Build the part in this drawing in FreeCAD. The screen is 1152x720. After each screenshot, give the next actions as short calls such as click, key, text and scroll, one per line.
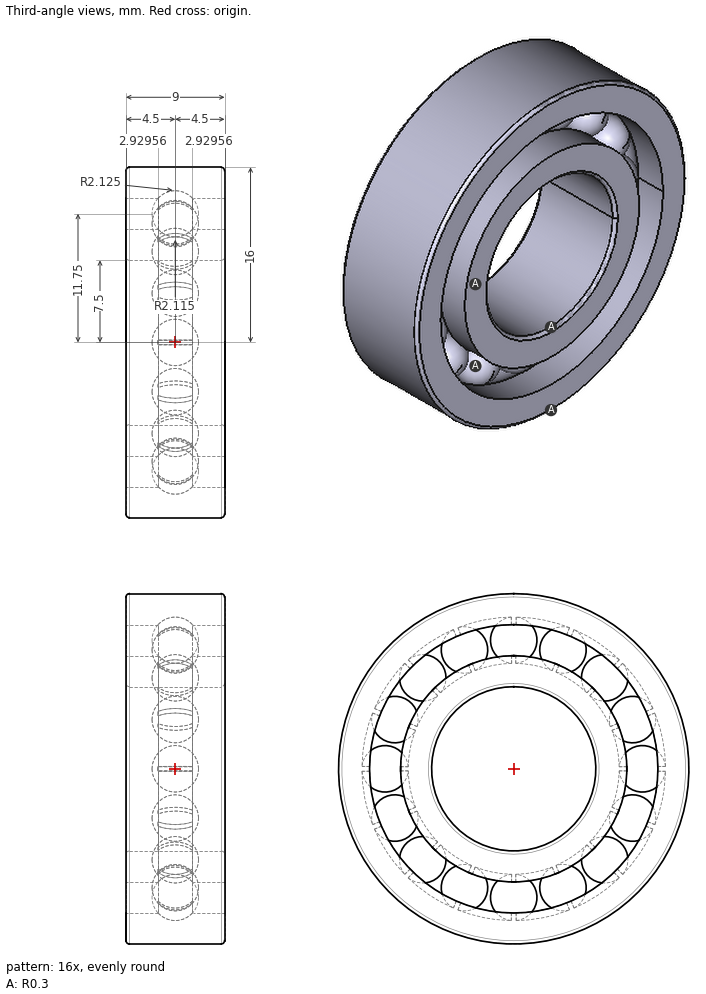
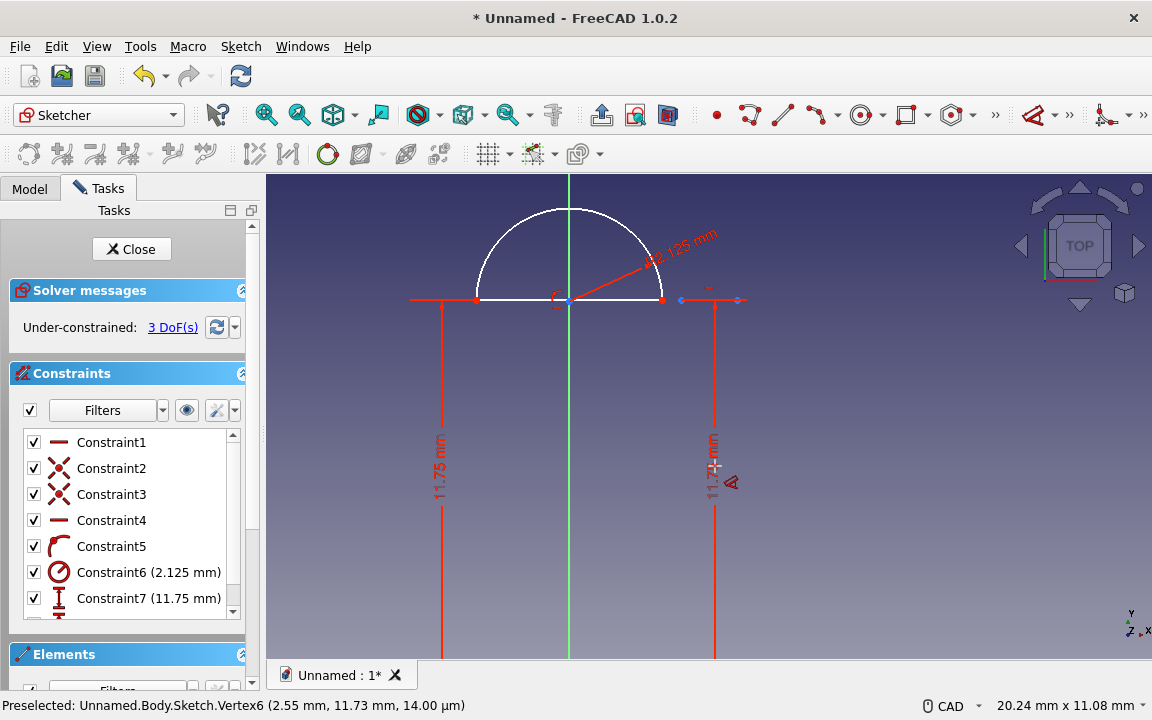
click(569, 302)
click(535, 466)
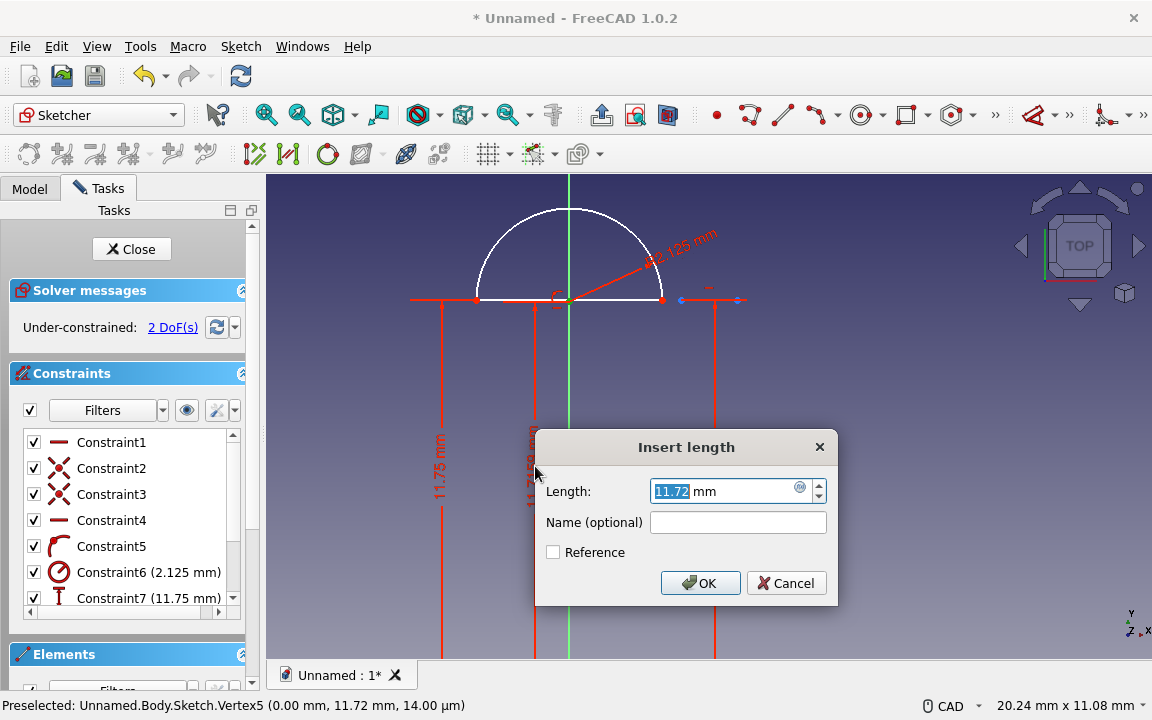
text(11.75)
key(Return)
key(Escape)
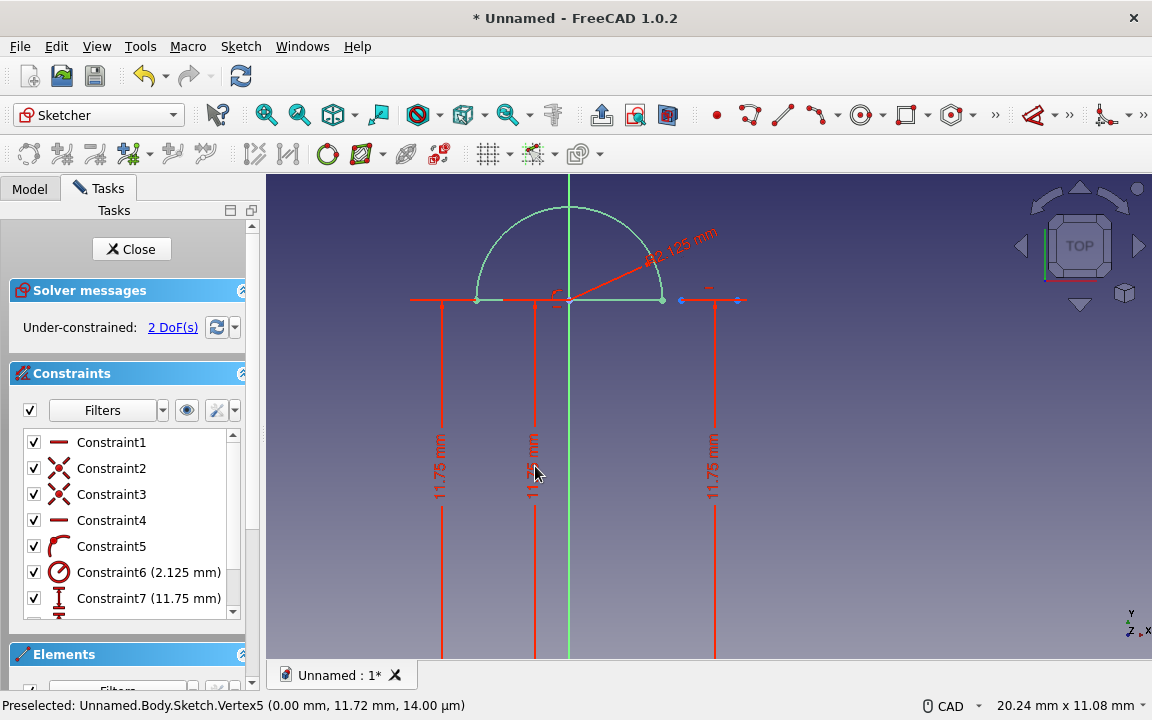
click(132, 249)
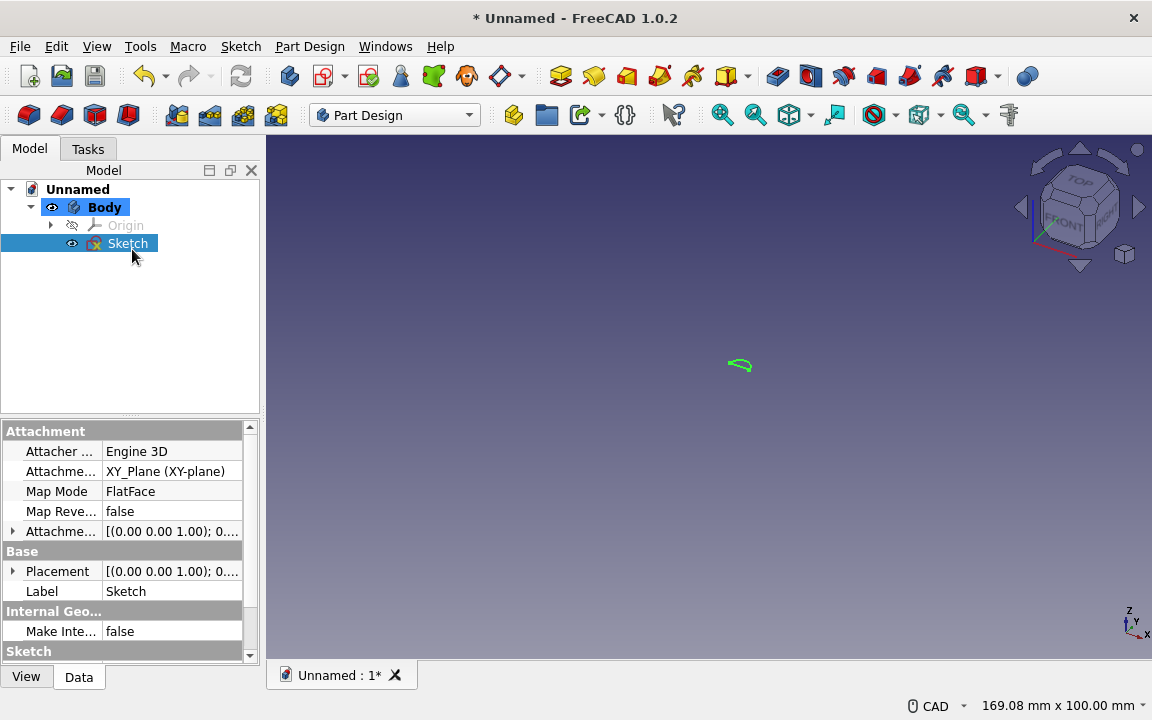
click(594, 76)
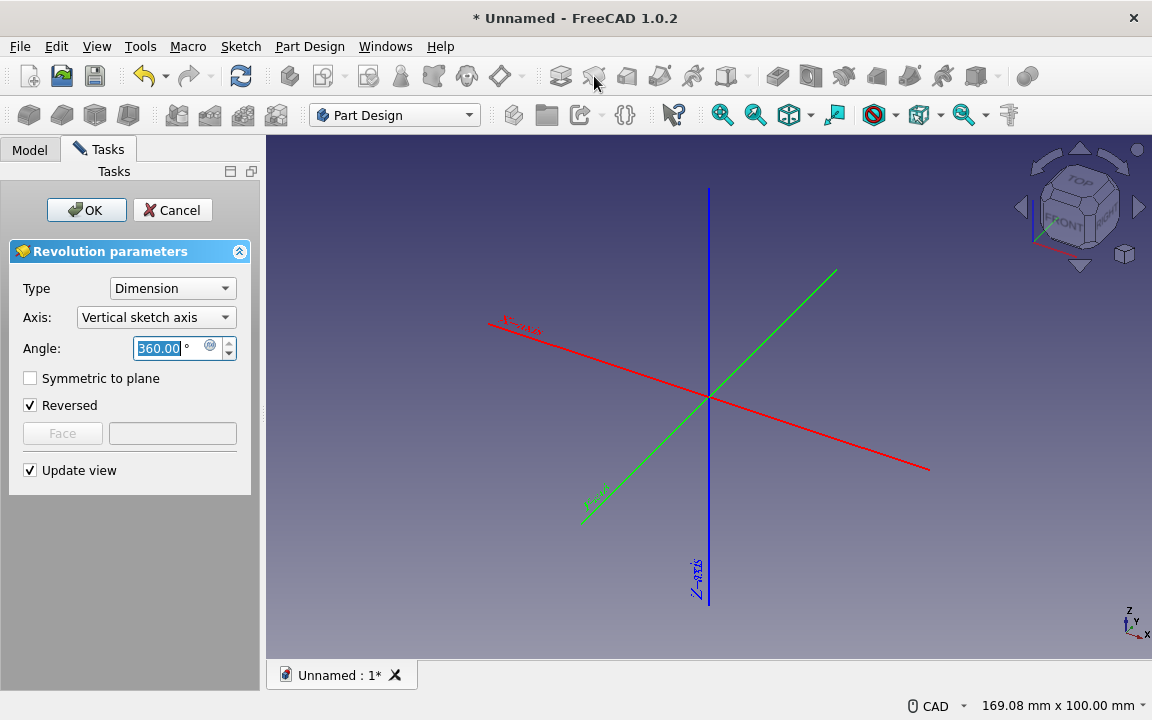
click(157, 318)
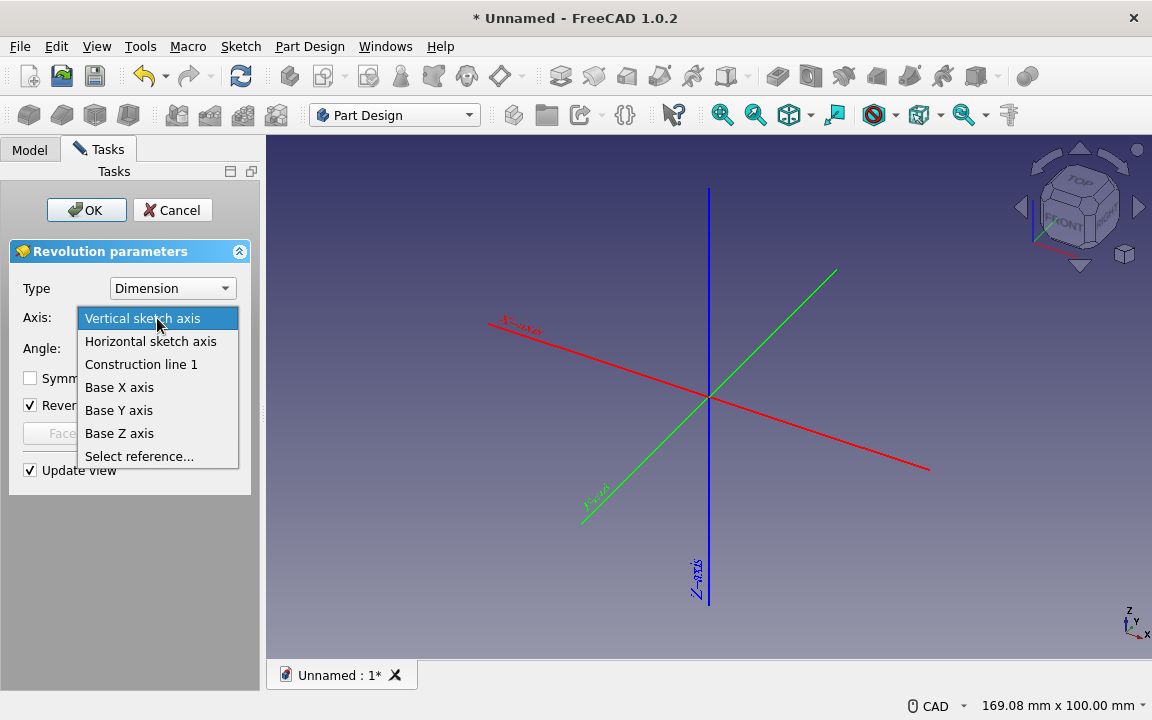
click(156, 364)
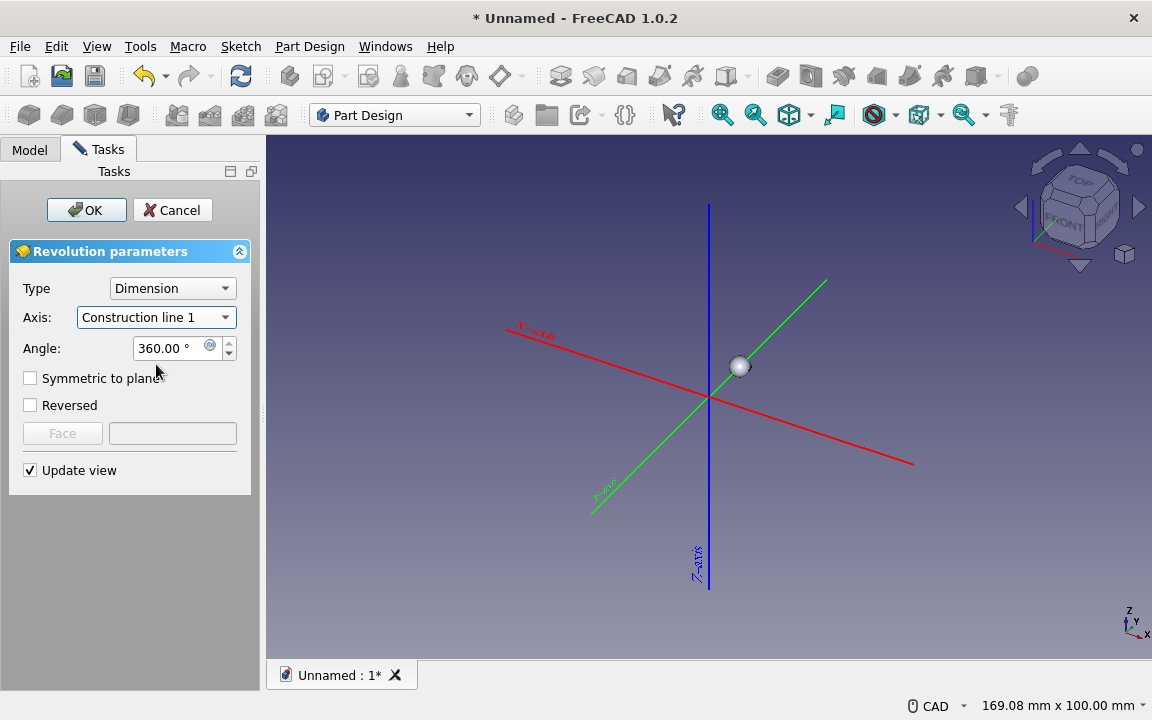
click(87, 210)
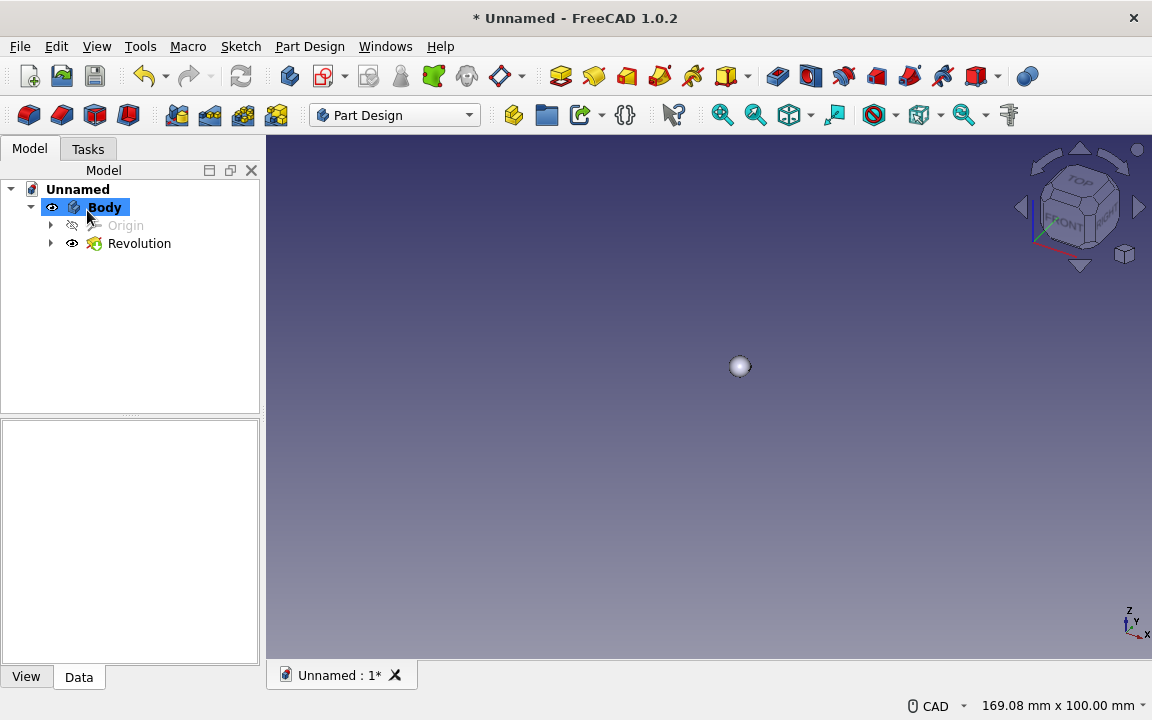
click(723, 116)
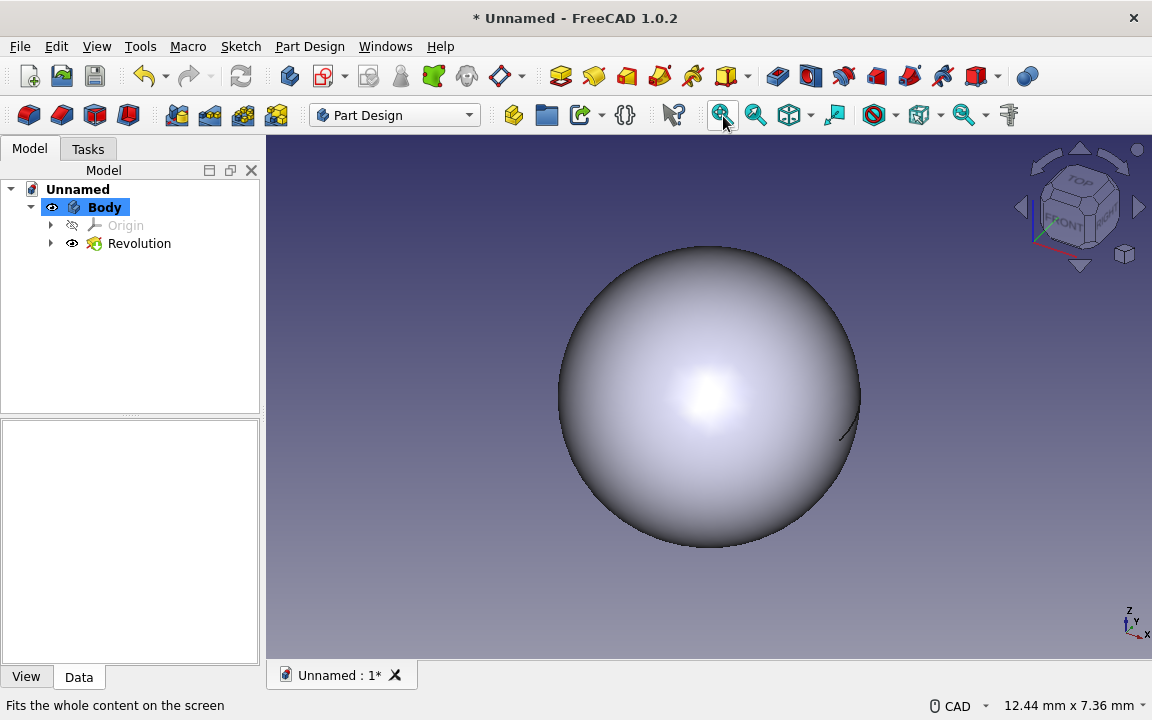
click(322, 76)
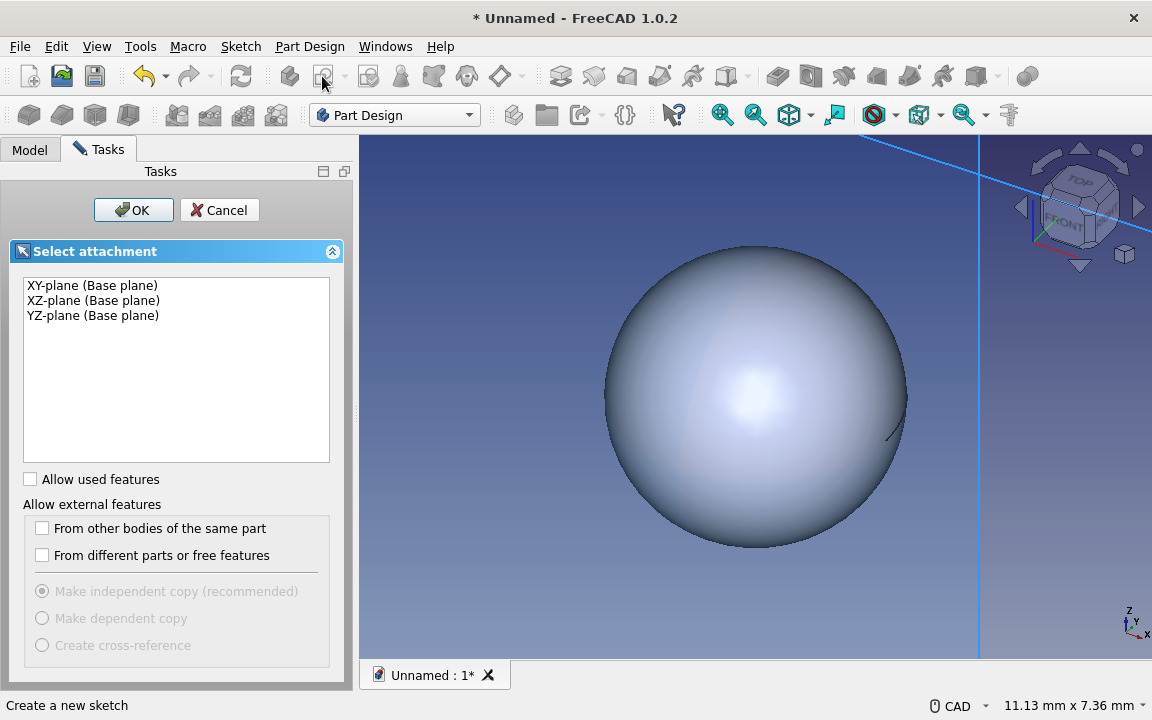
click(84, 286)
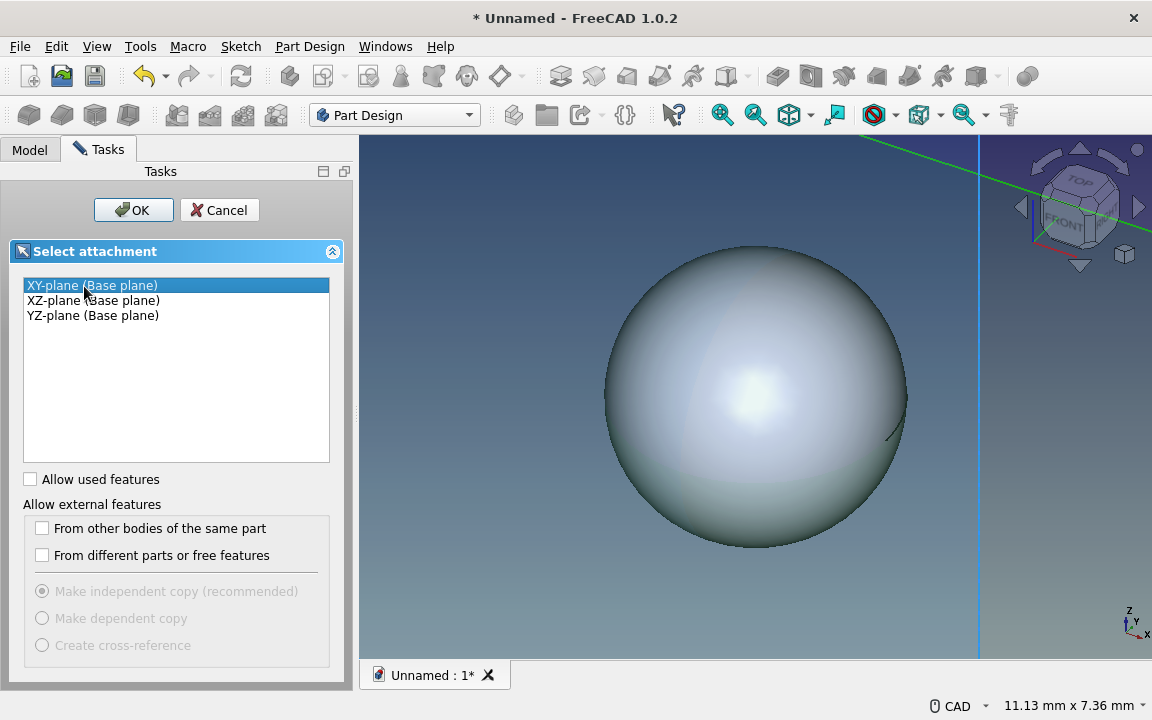
click(134, 210)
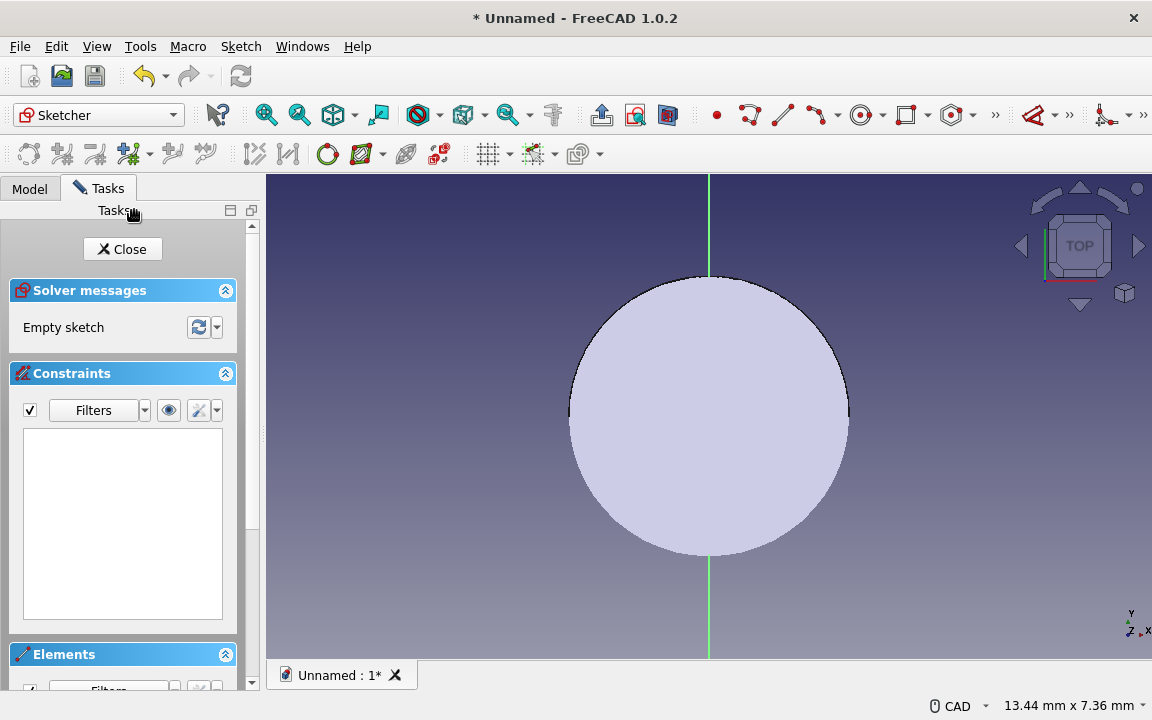
click(668, 116)